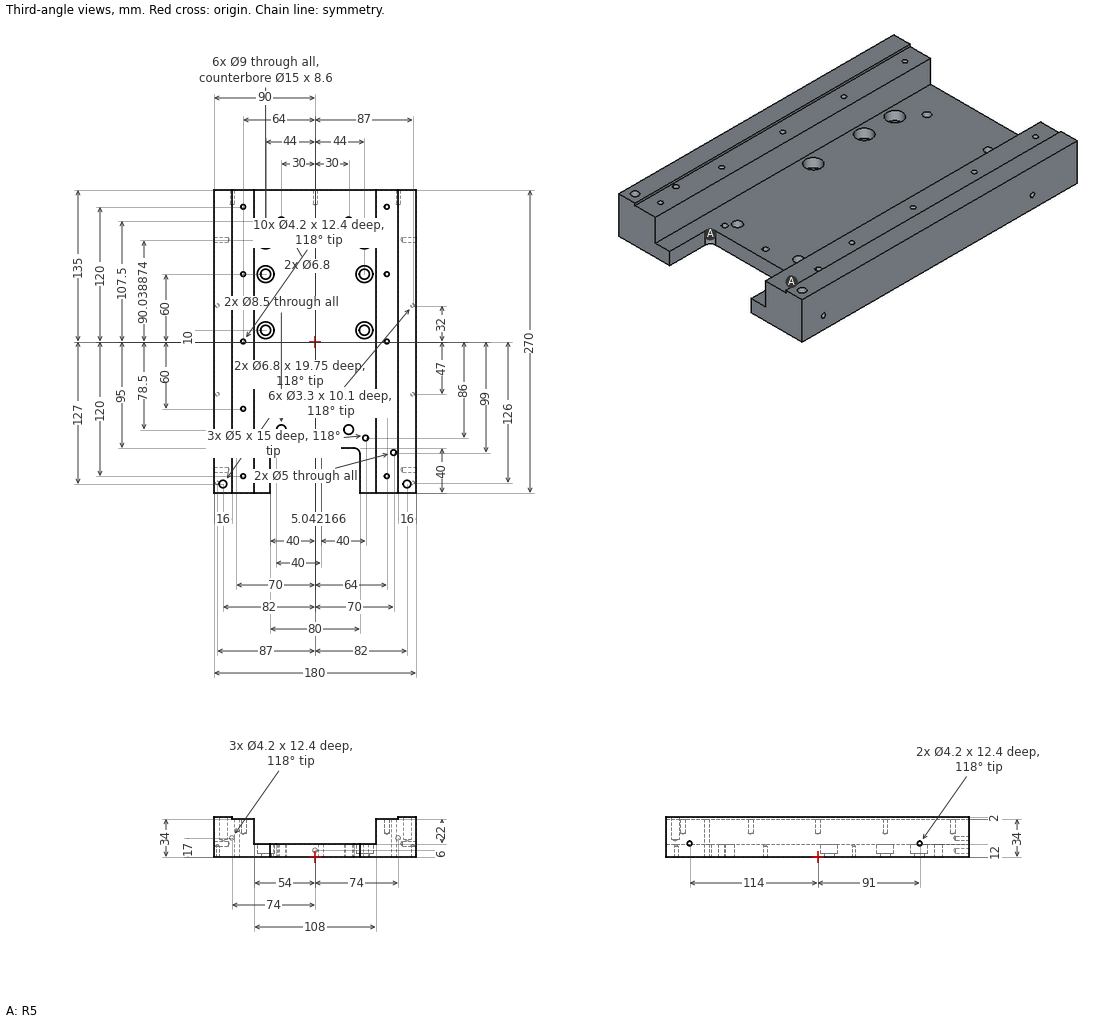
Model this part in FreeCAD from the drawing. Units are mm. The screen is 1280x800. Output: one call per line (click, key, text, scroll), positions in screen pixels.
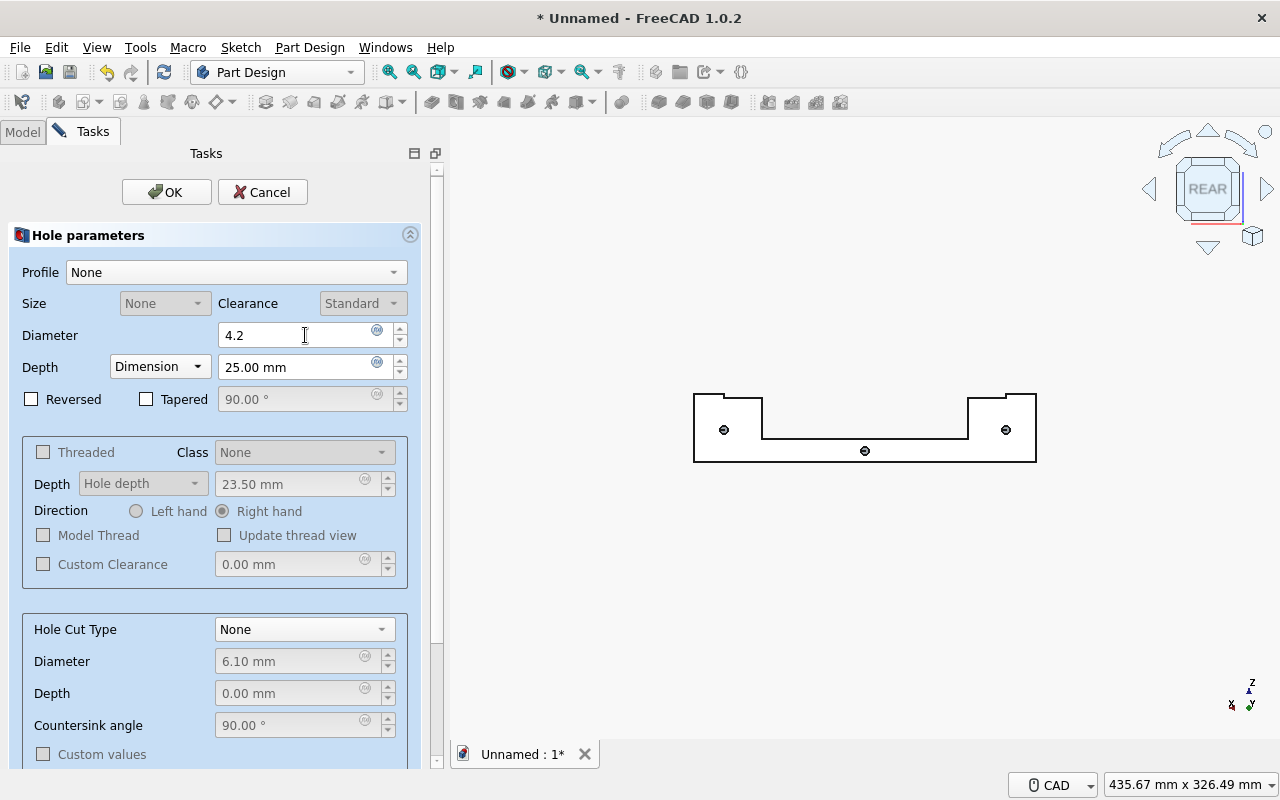
triple_click(305, 367)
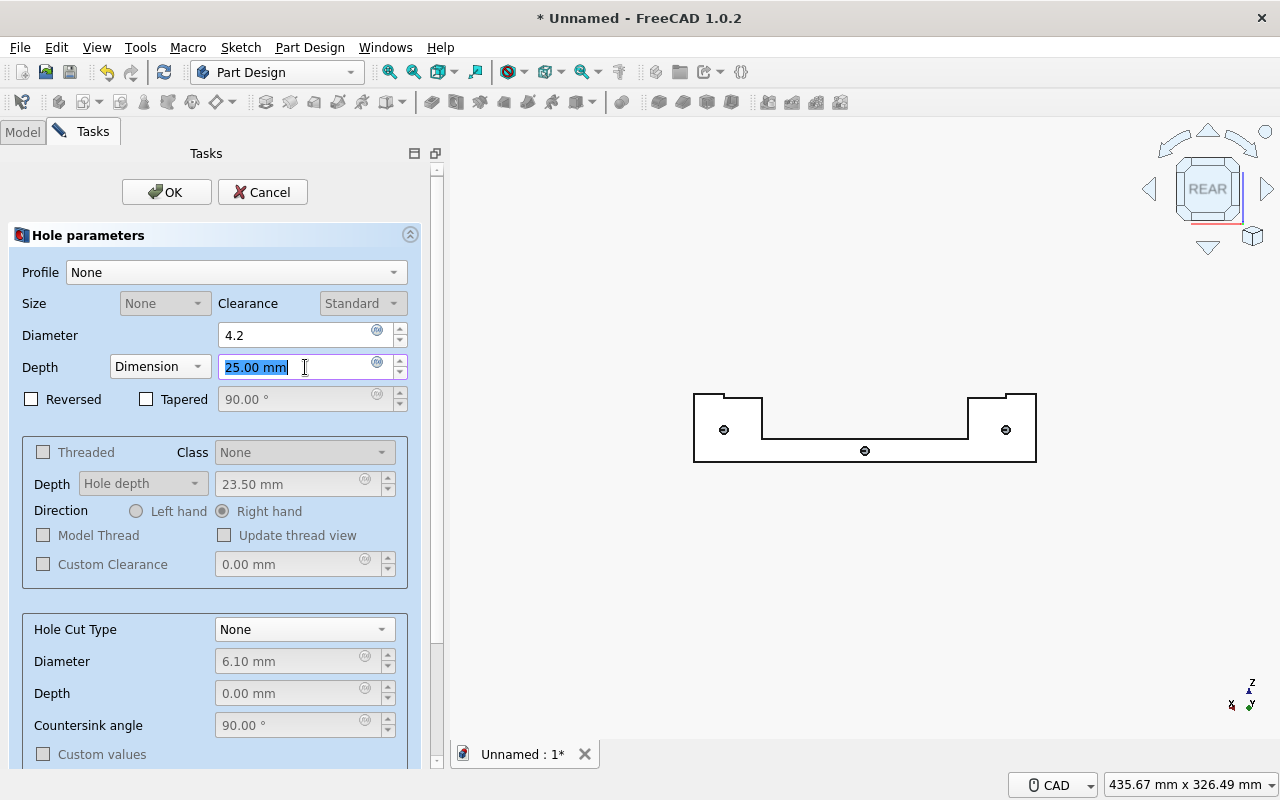
text(12.4)
key(Tab)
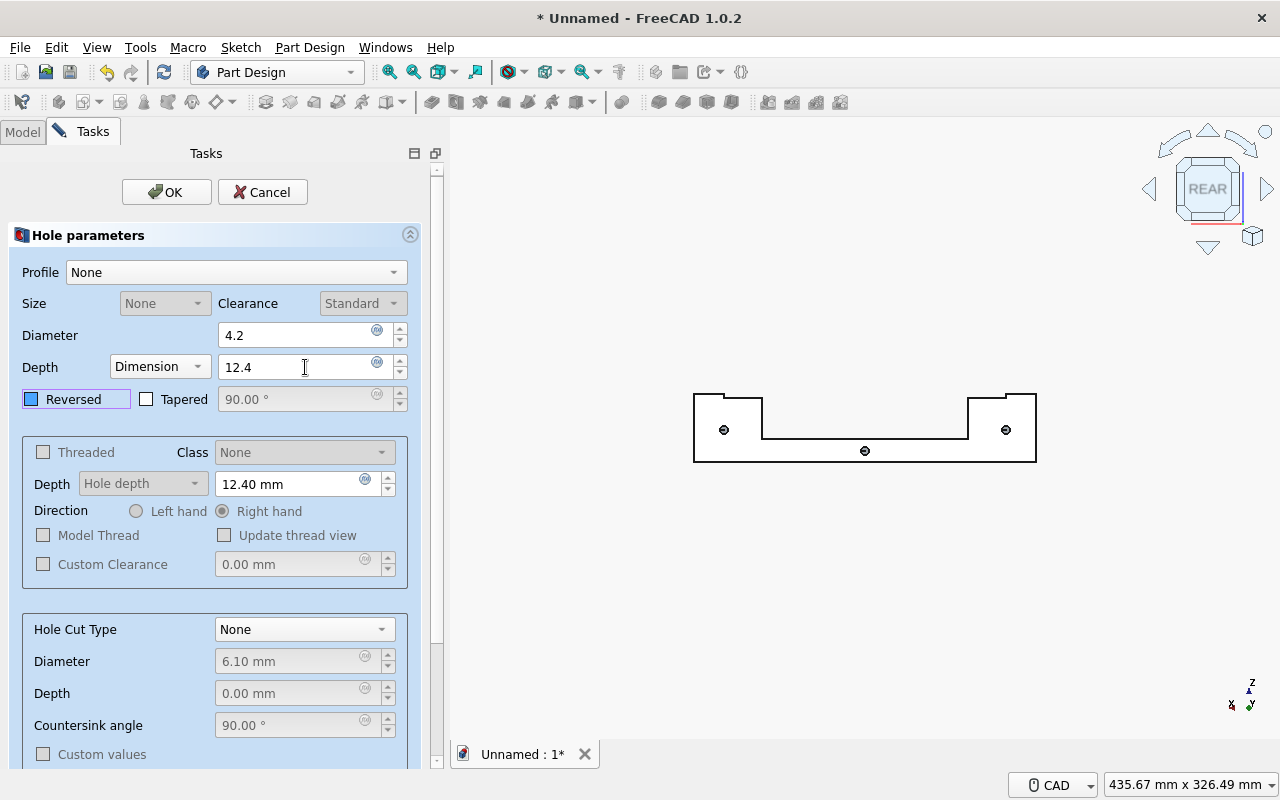
click(167, 192)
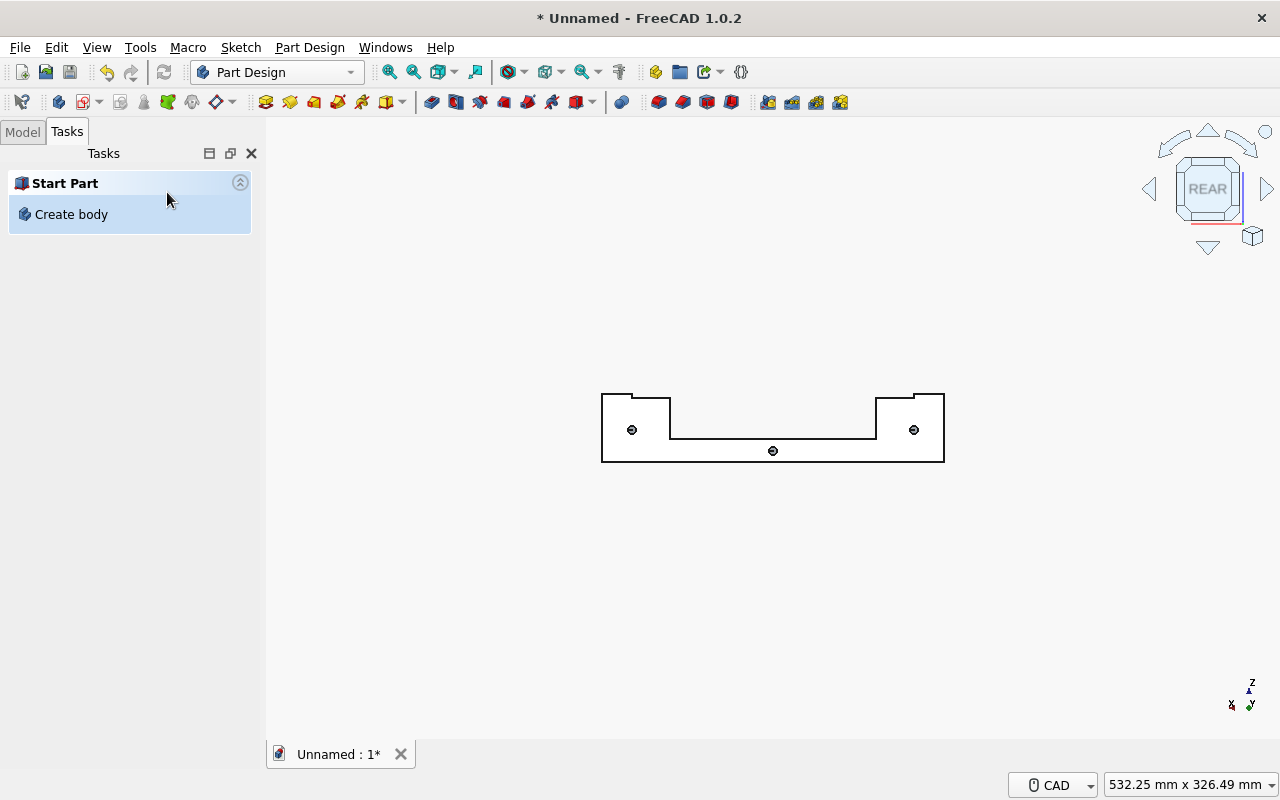
click(390, 72)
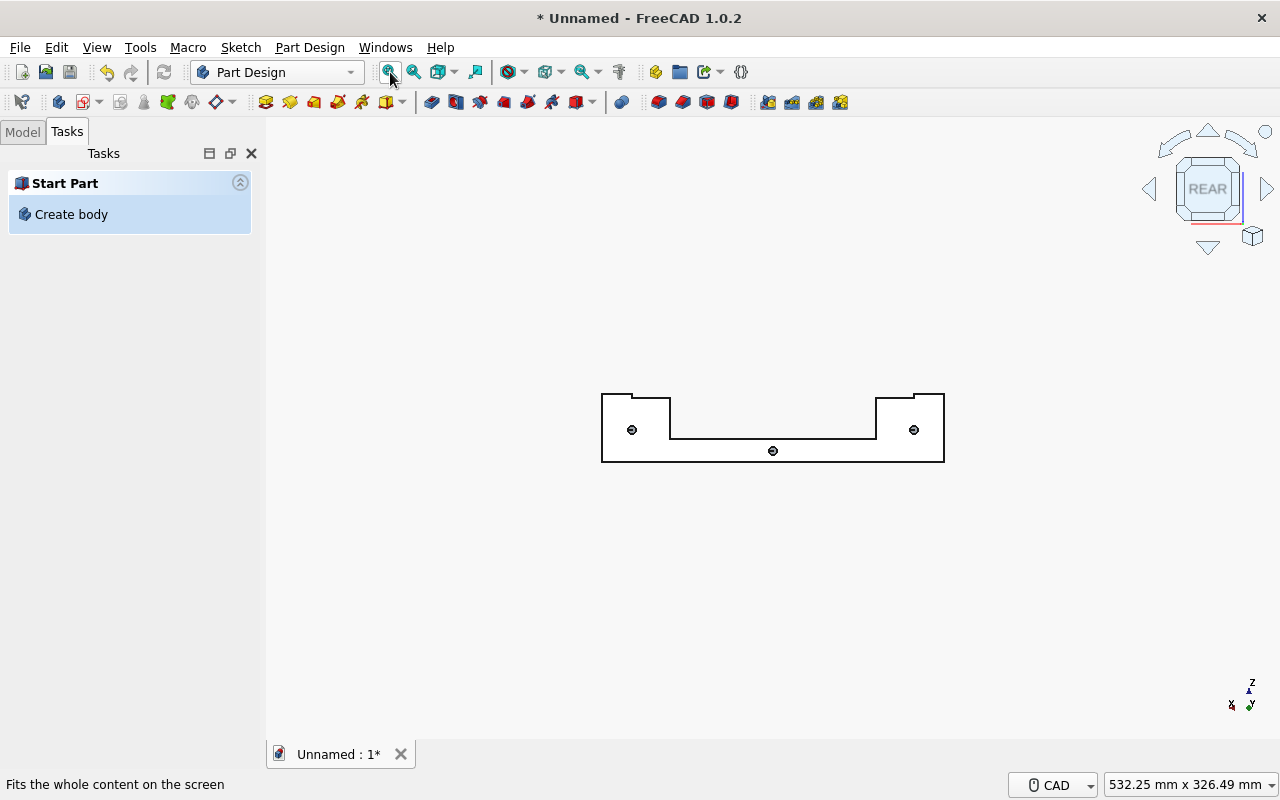
click(84, 102)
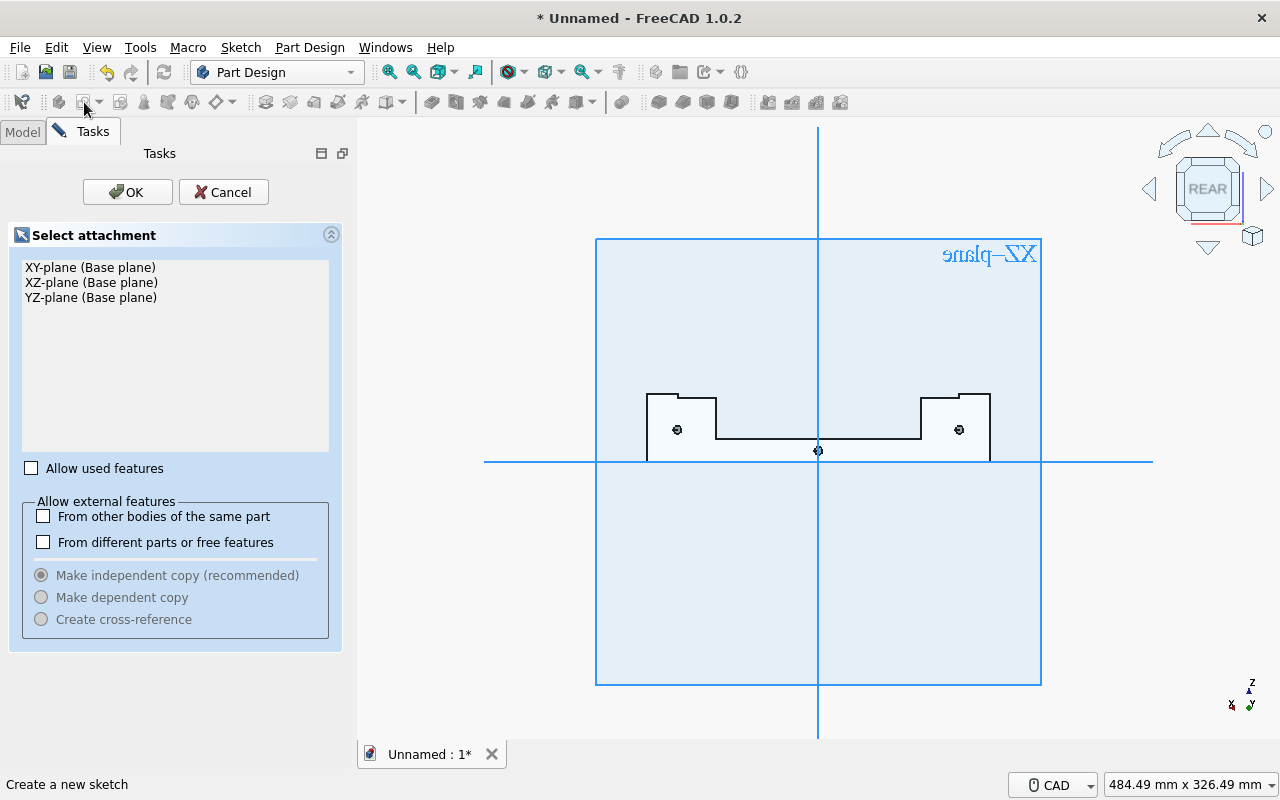
click(82, 268)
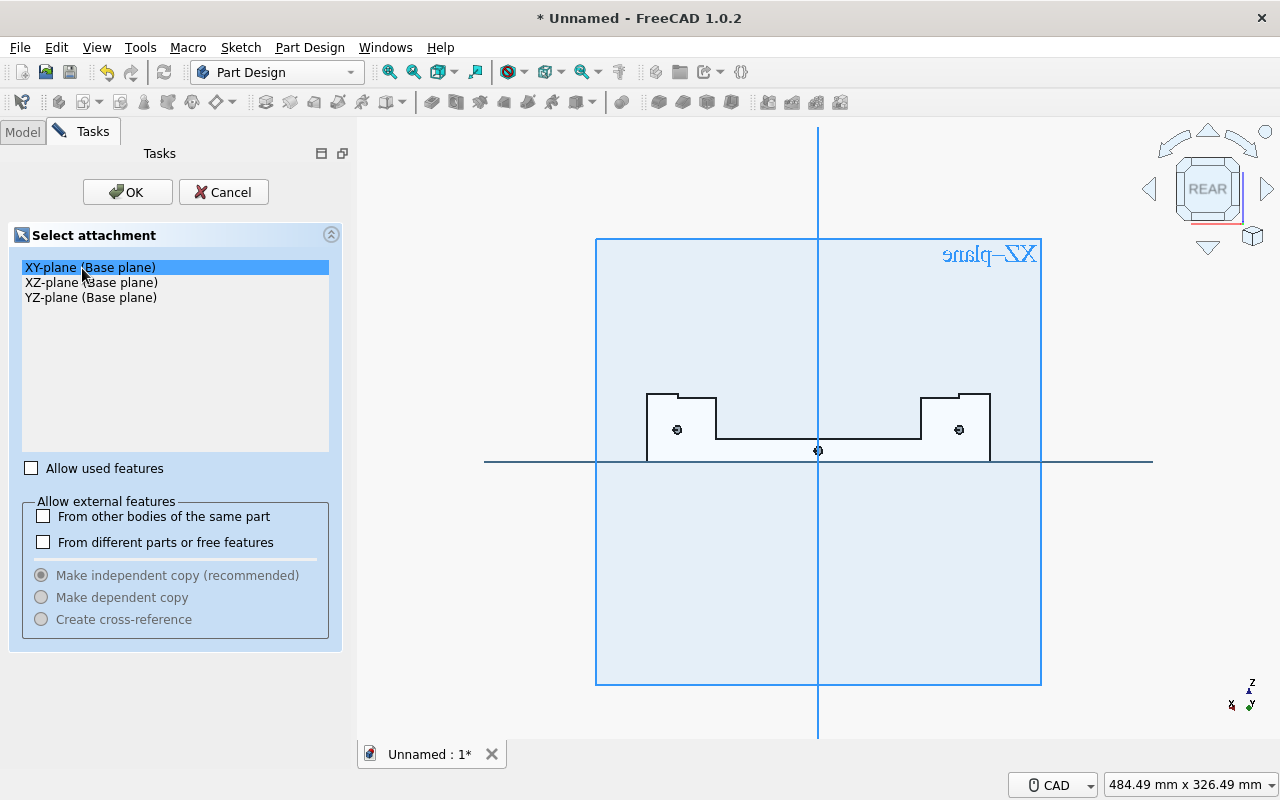
click(128, 192)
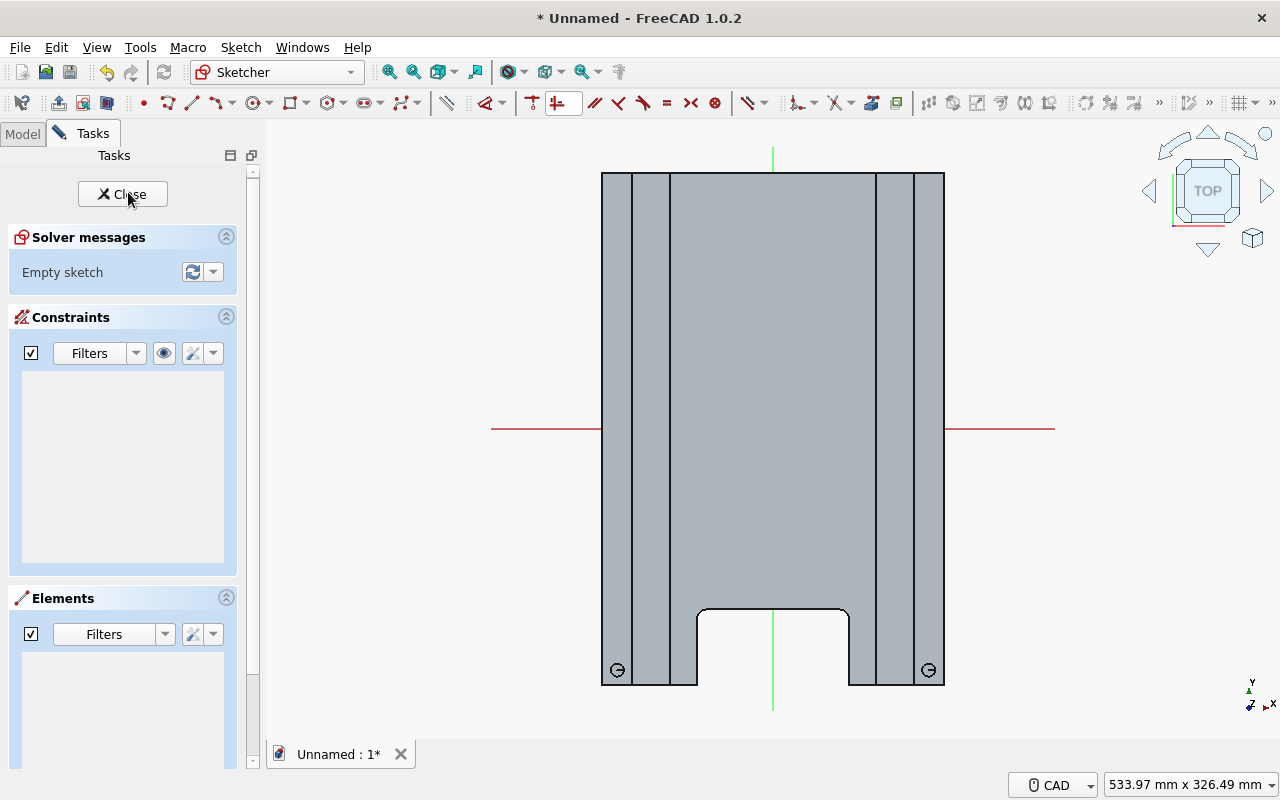
key(q)
key(s)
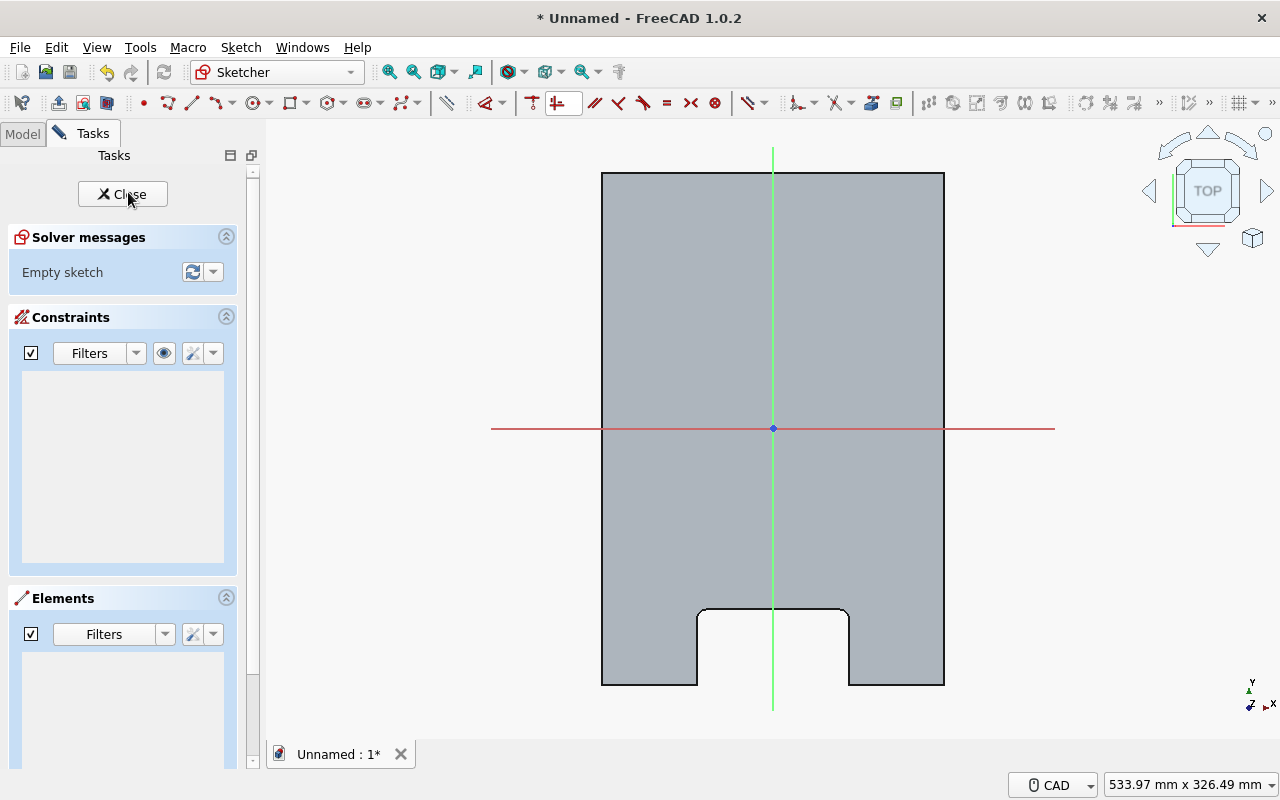
scroll(846, 582, up, 4)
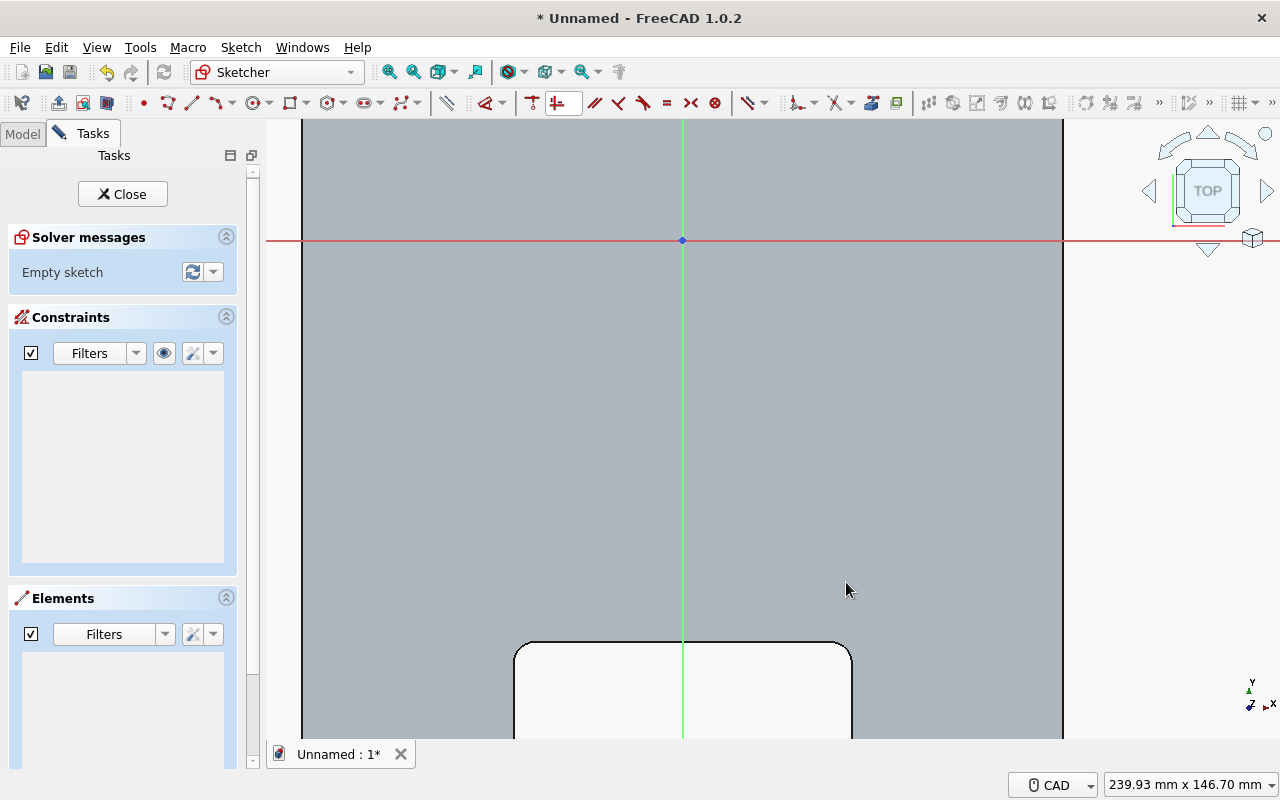
click(254, 104)